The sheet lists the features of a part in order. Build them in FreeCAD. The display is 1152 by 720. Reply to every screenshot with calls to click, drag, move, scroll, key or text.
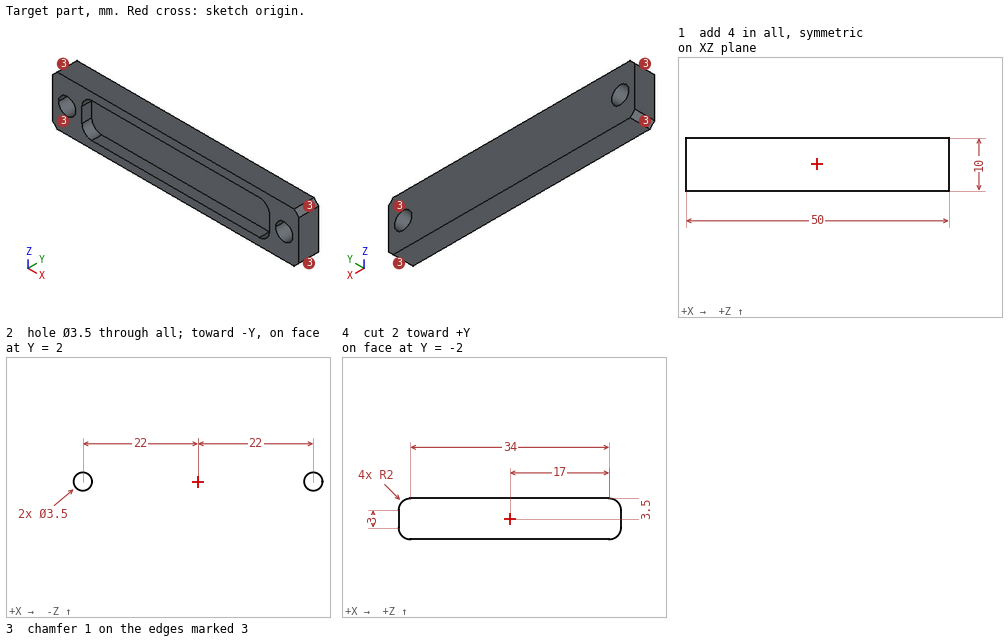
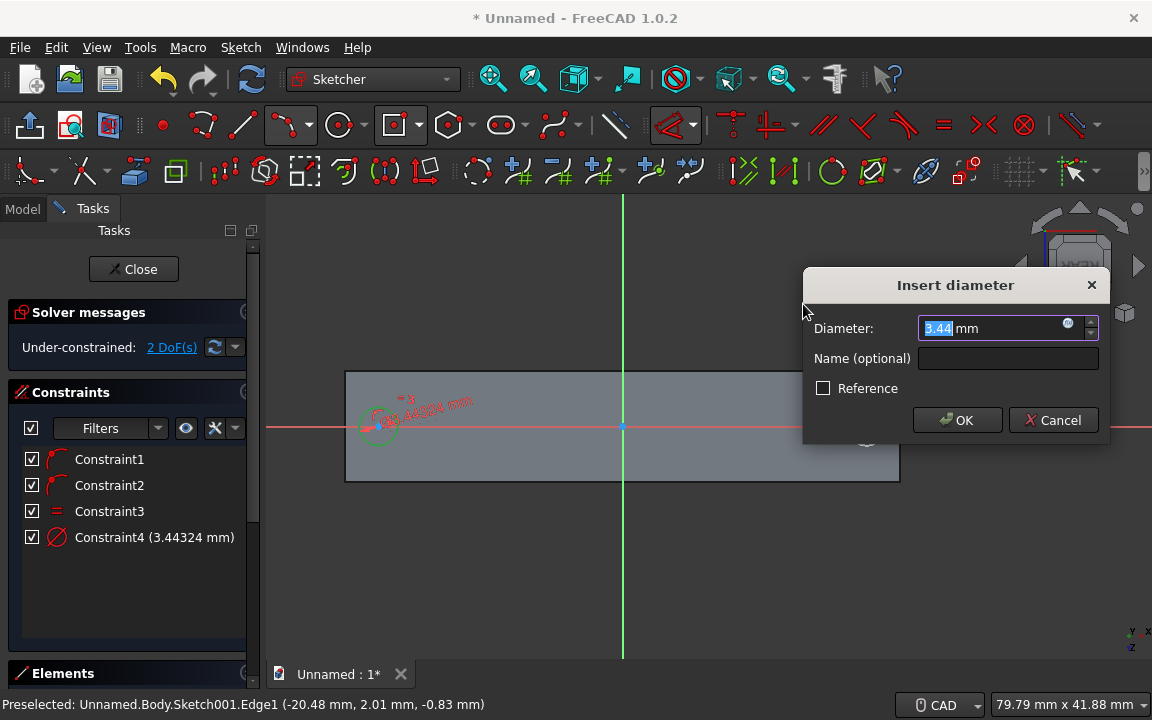
text(3.5)
key(Return)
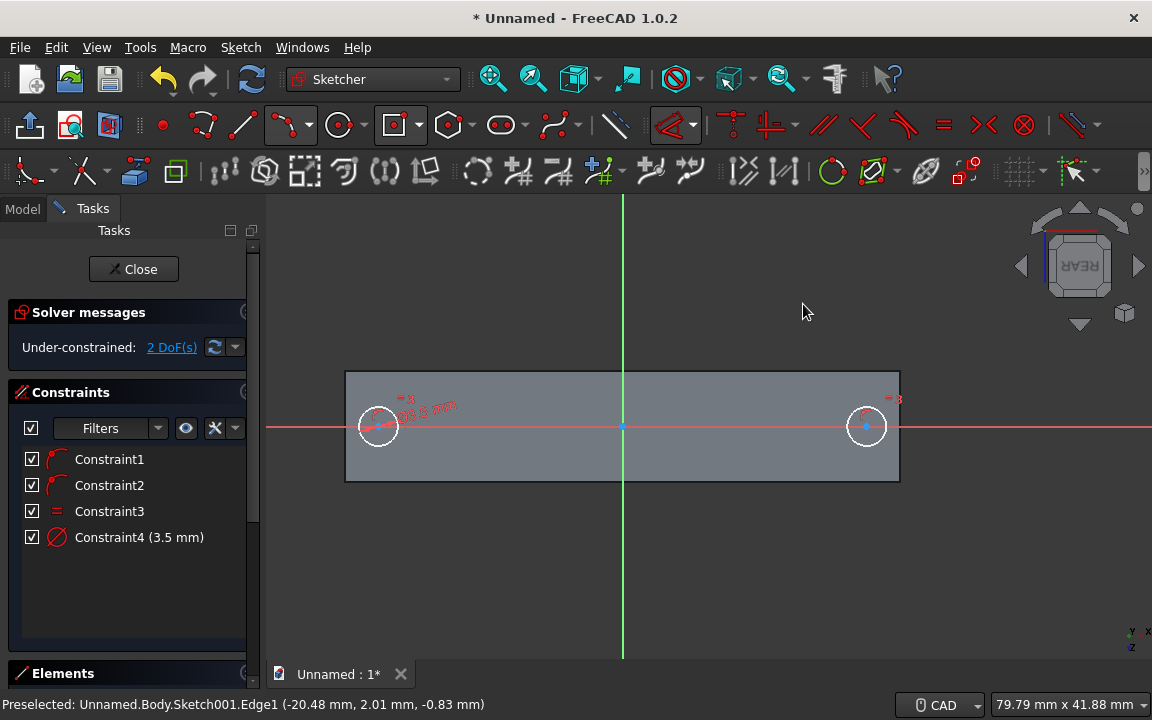
click(379, 427)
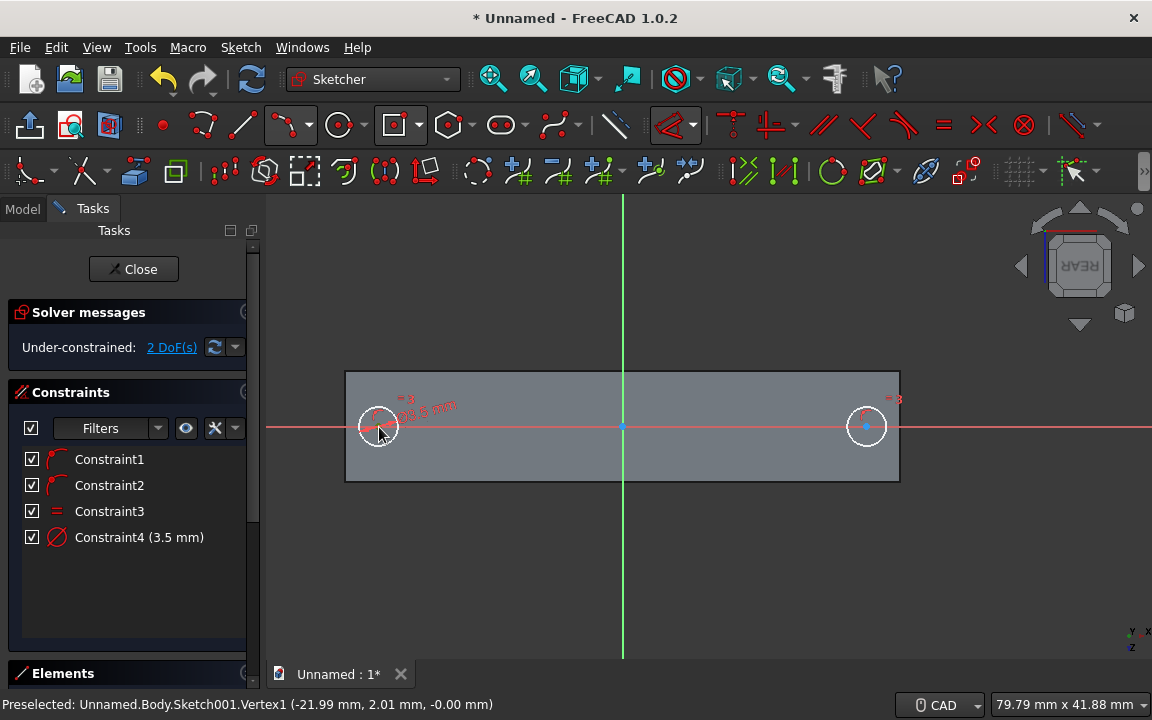
click(696, 126)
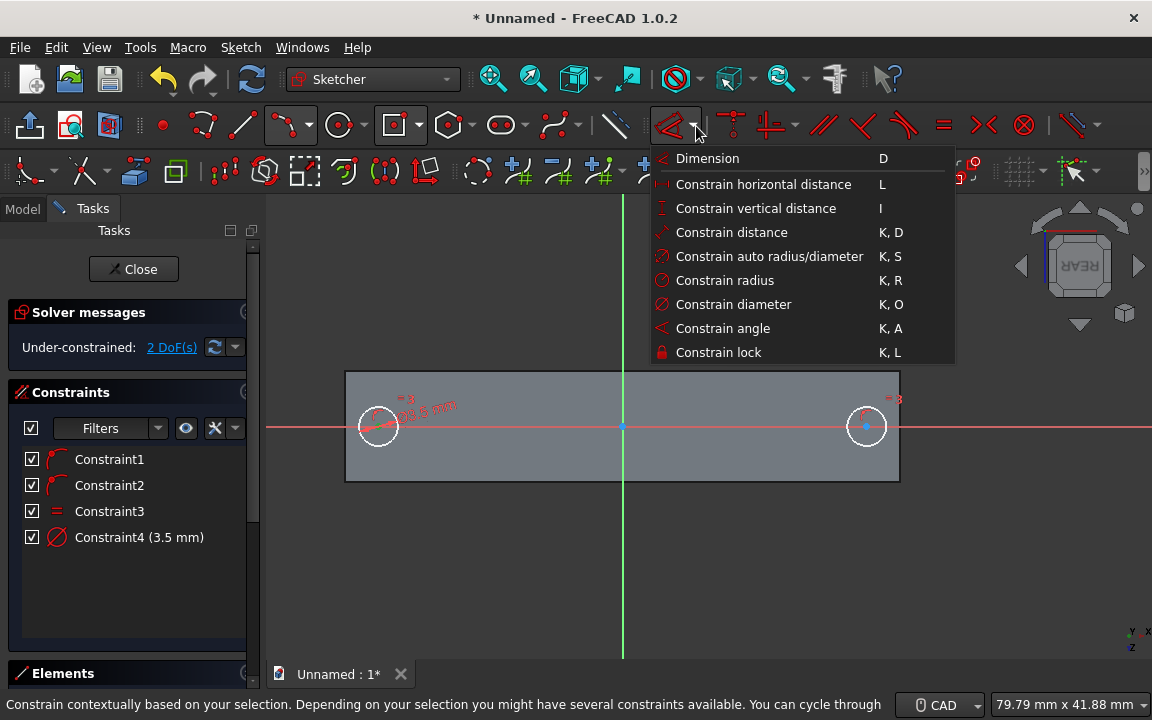
click(803, 184)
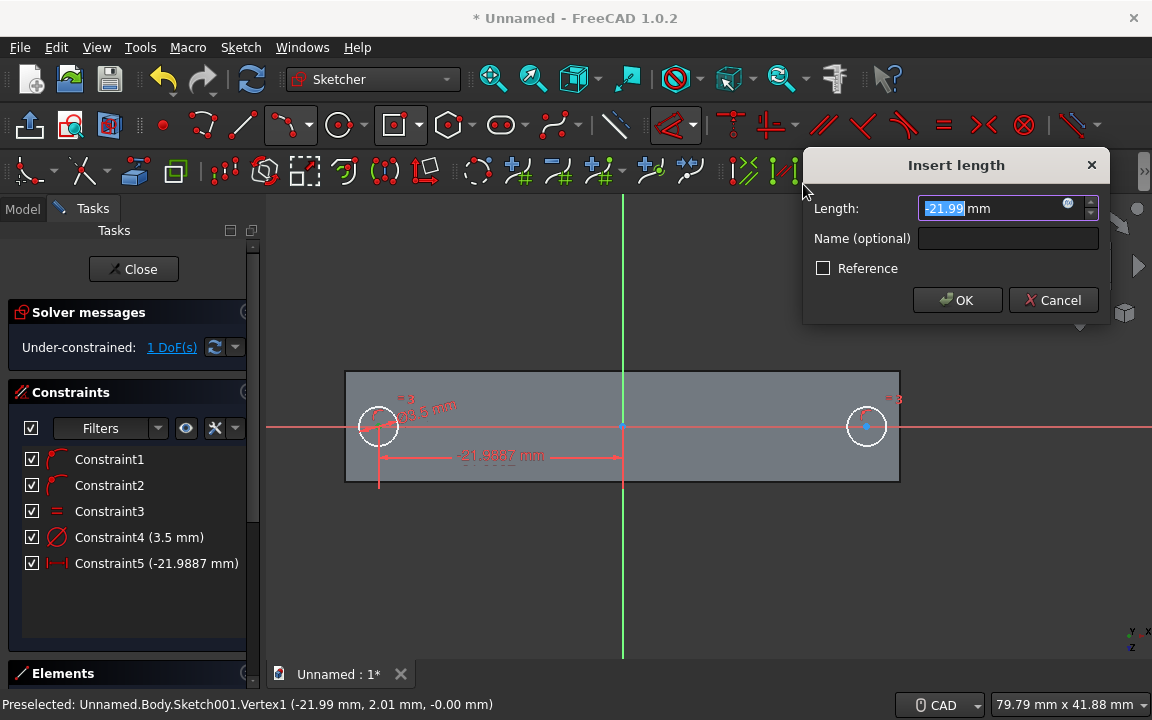
text(-22)
key(Return)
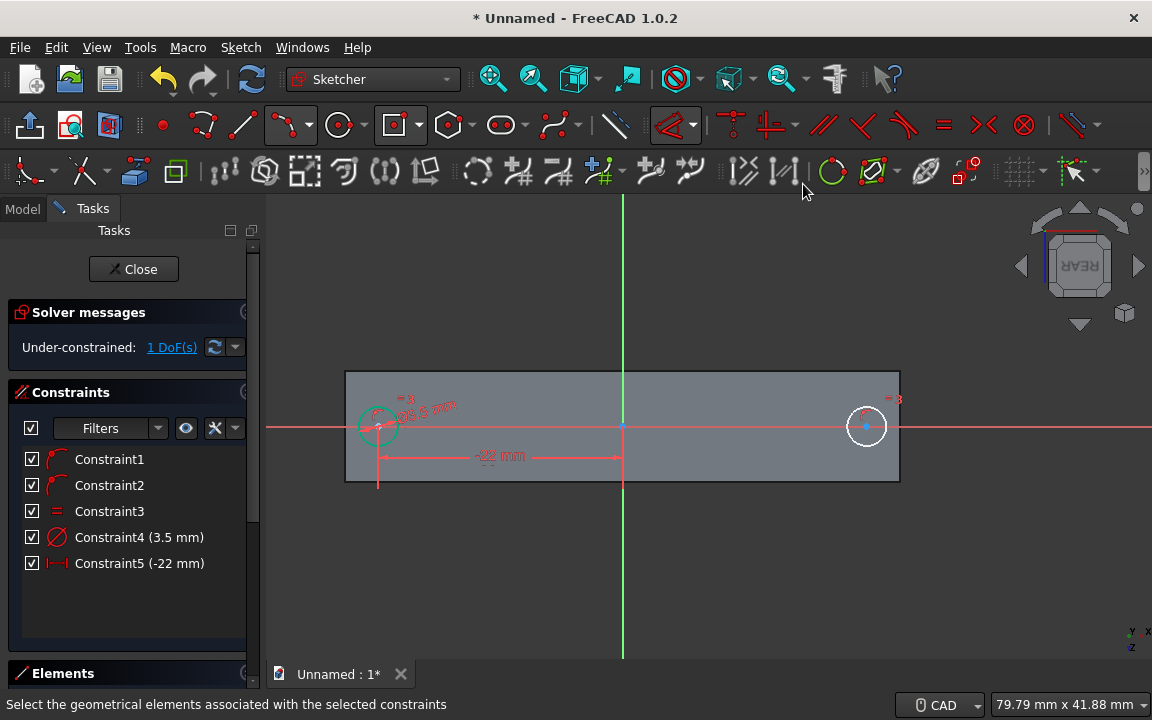
click(867, 427)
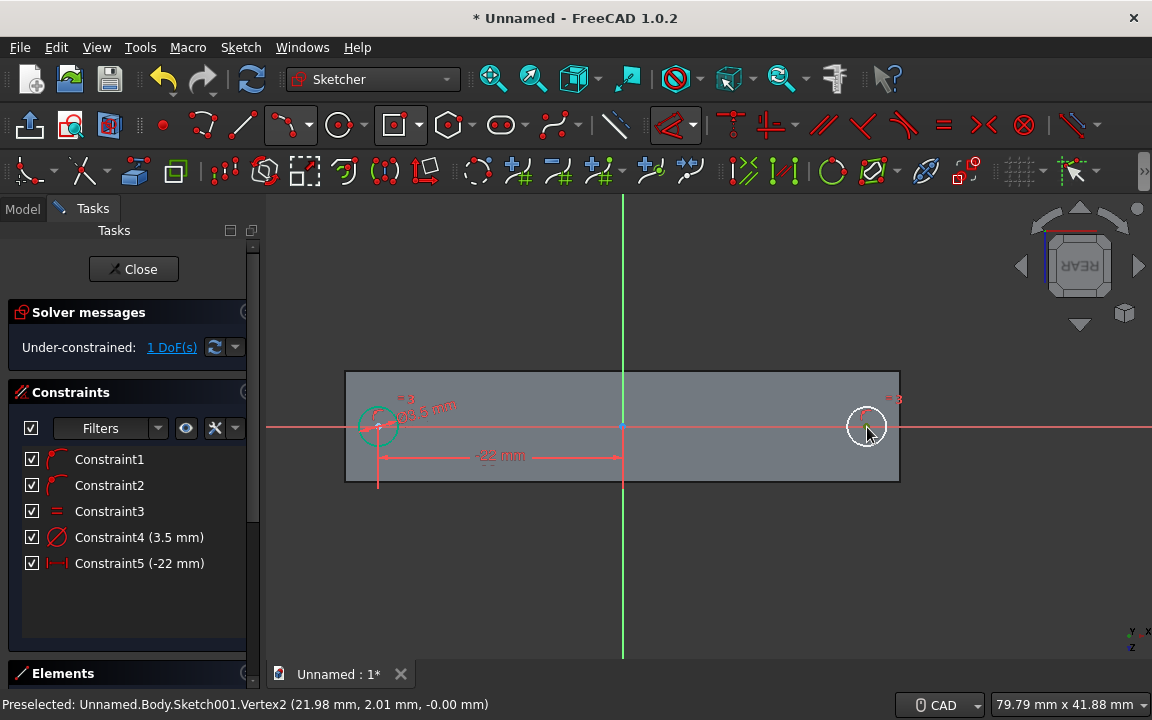
click(696, 126)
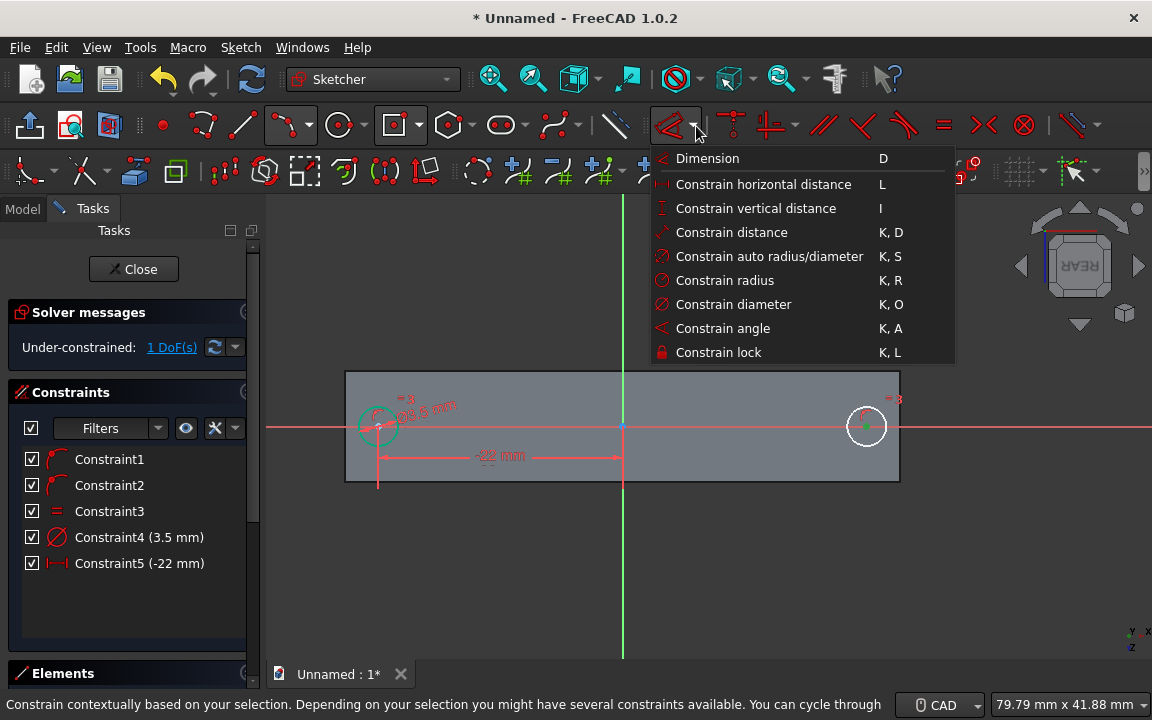
click(803, 184)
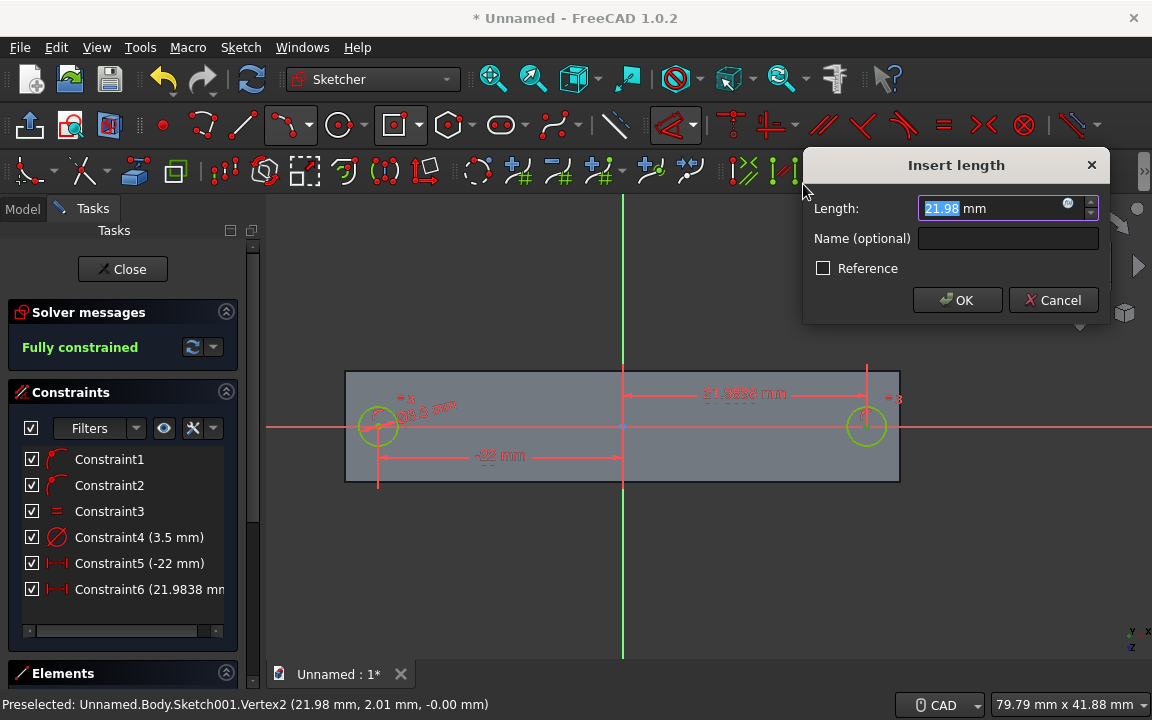
text(22)
key(Return)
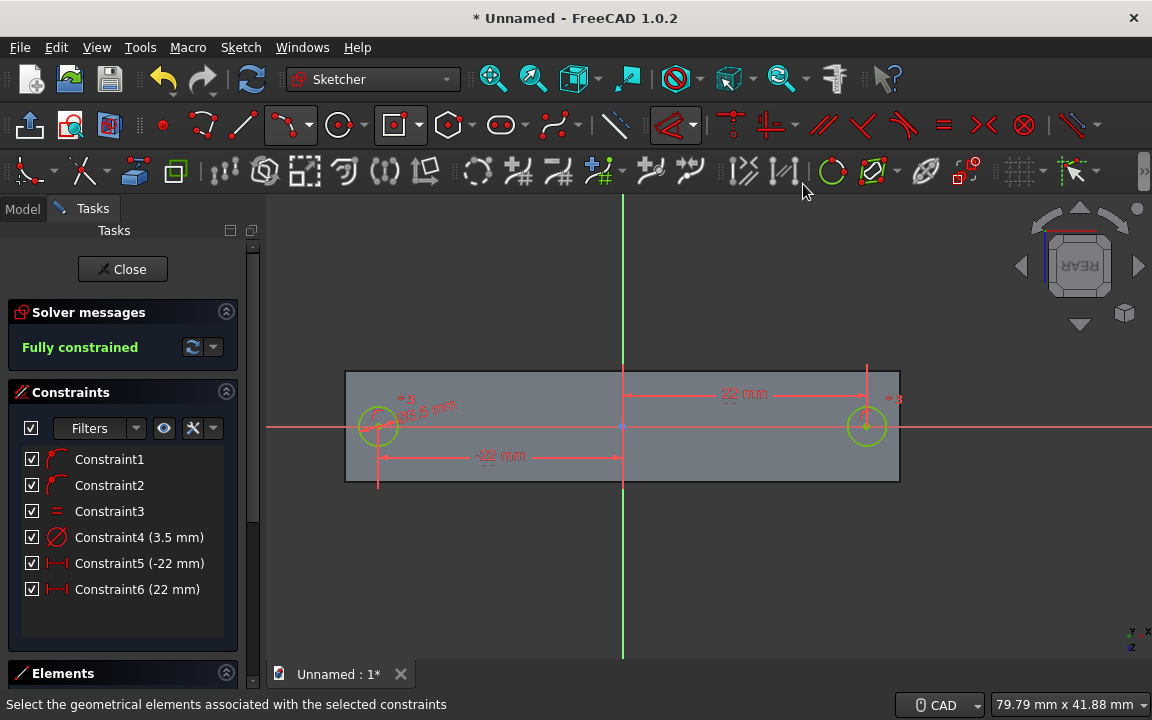
click(123, 269)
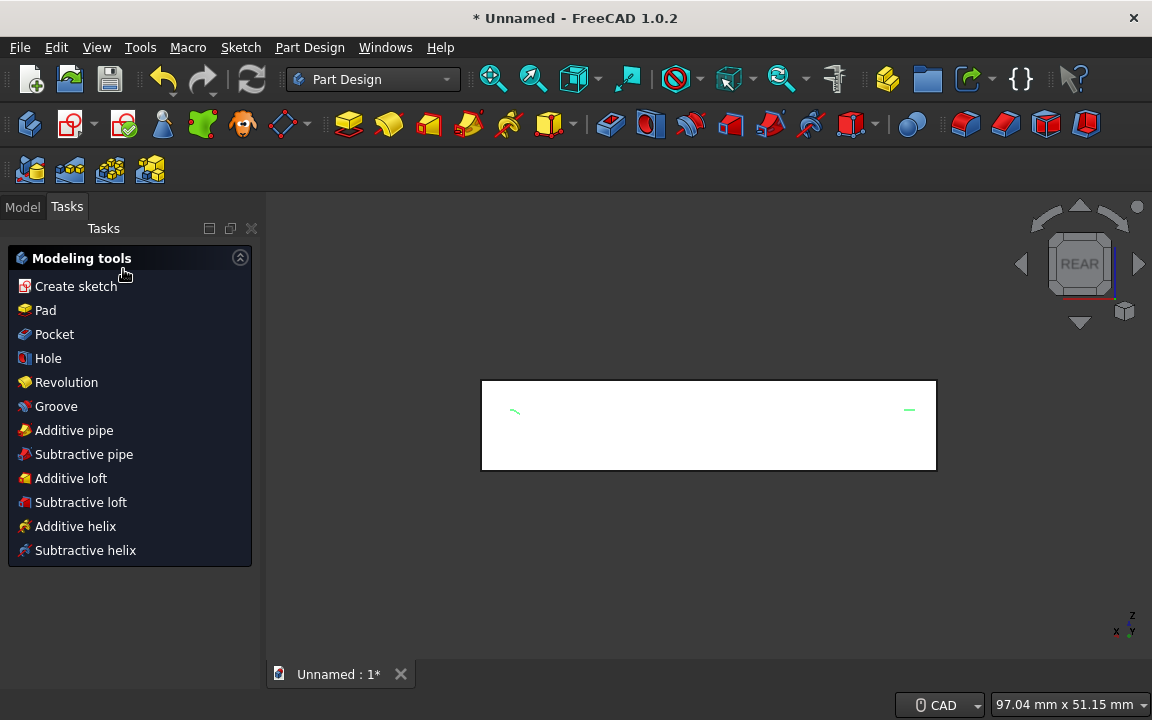
click(652, 124)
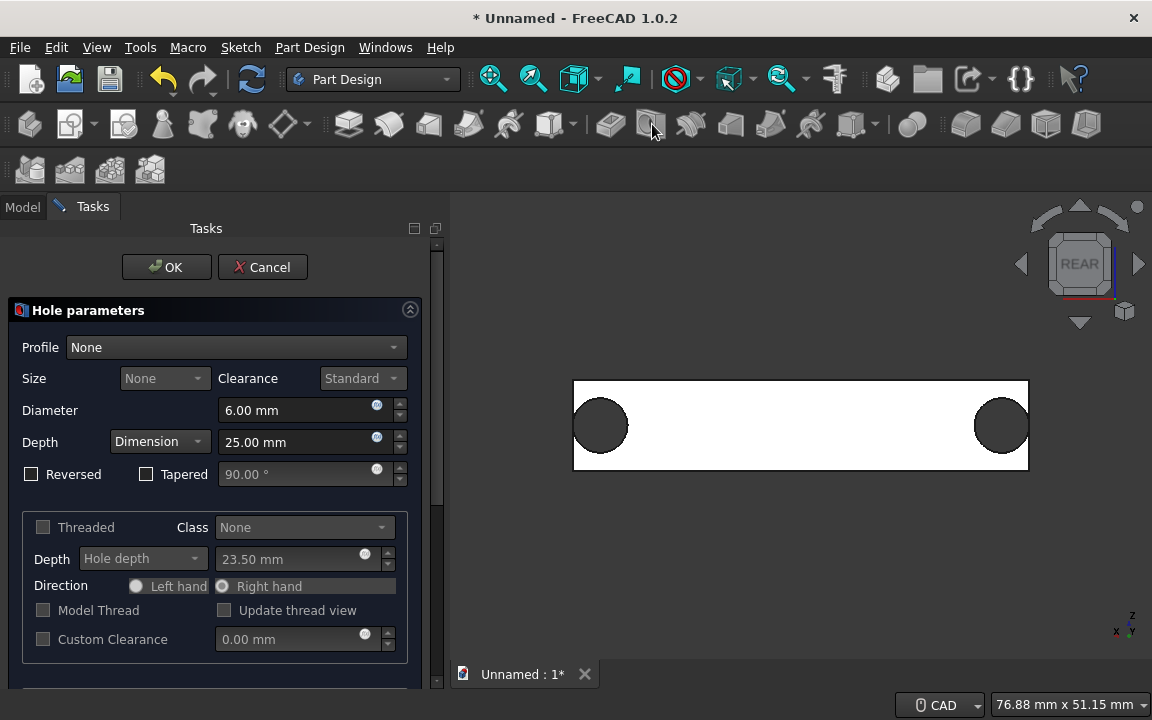
triple_click(305, 410)